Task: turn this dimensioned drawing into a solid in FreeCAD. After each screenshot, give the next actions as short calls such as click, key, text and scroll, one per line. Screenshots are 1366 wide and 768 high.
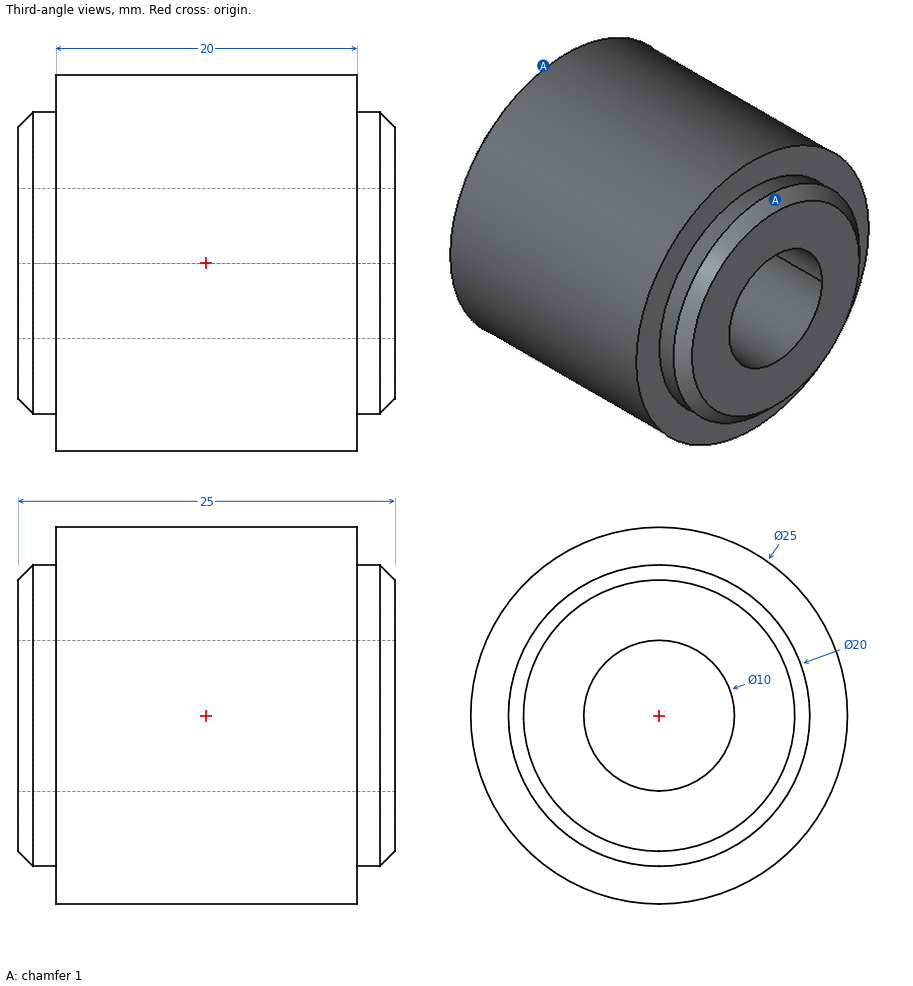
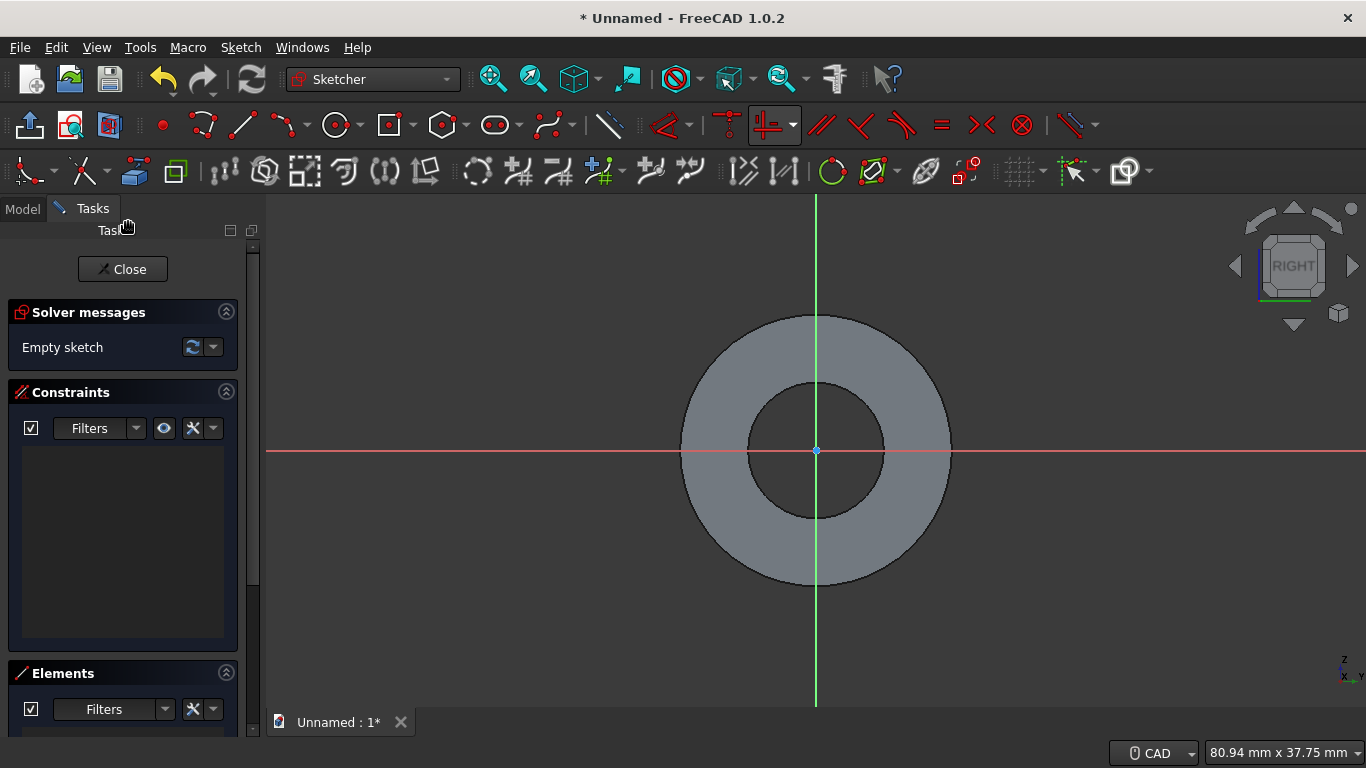
key(g)
key(c)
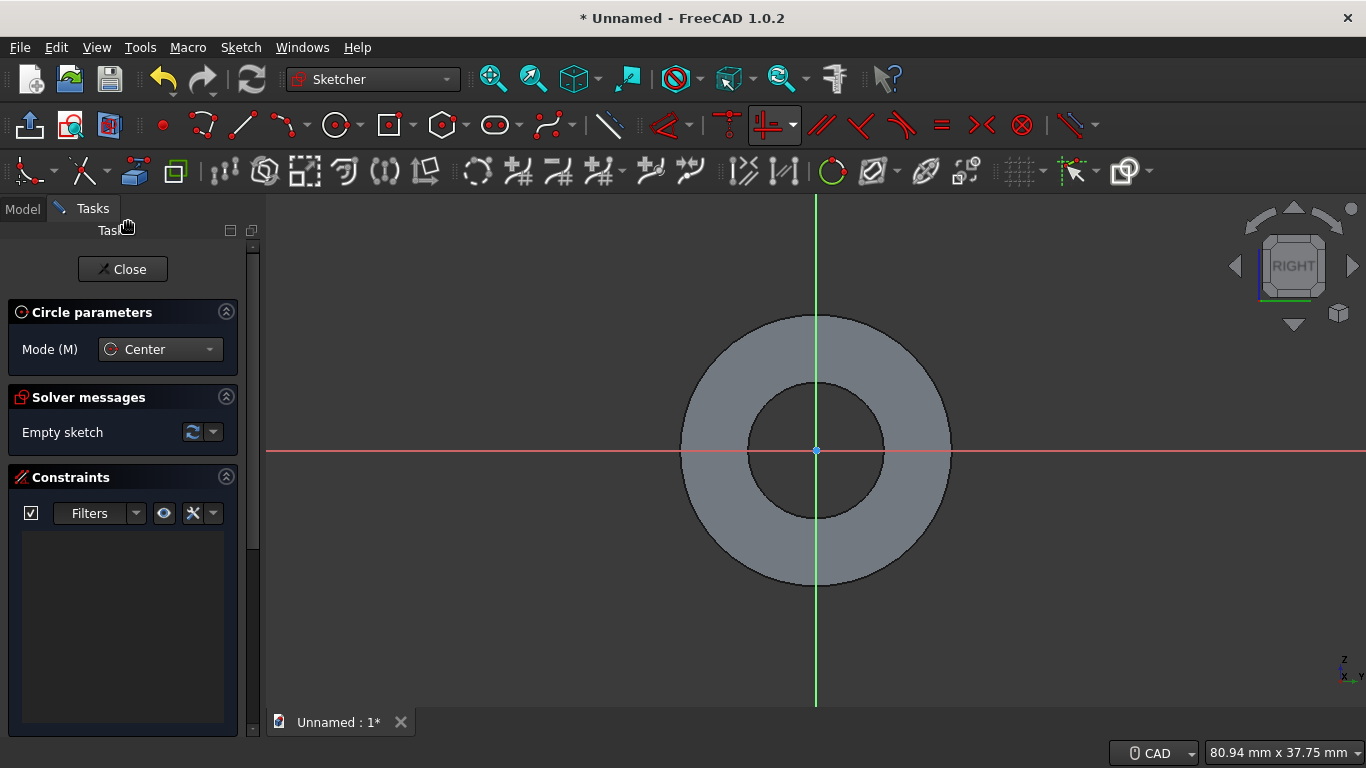
click(816, 450)
move(936, 330)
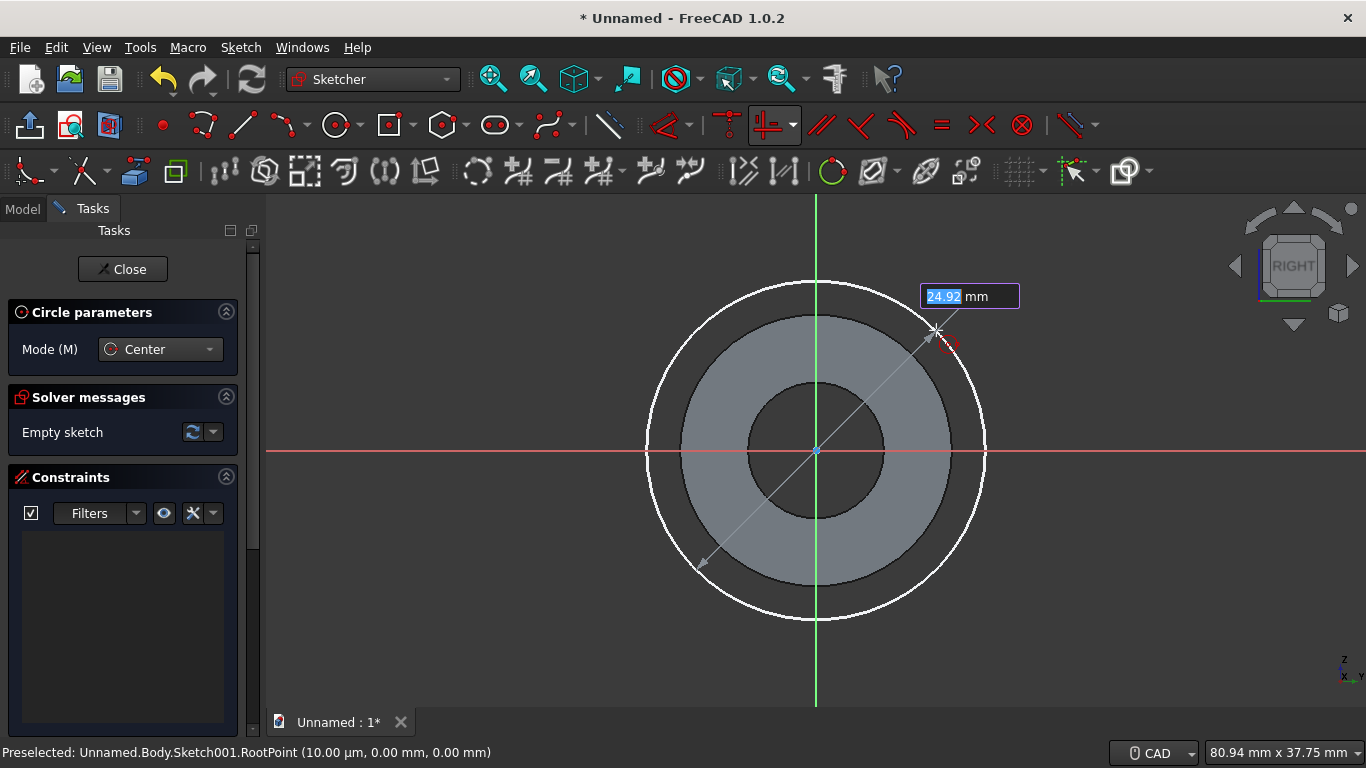
text(25)
key(Return)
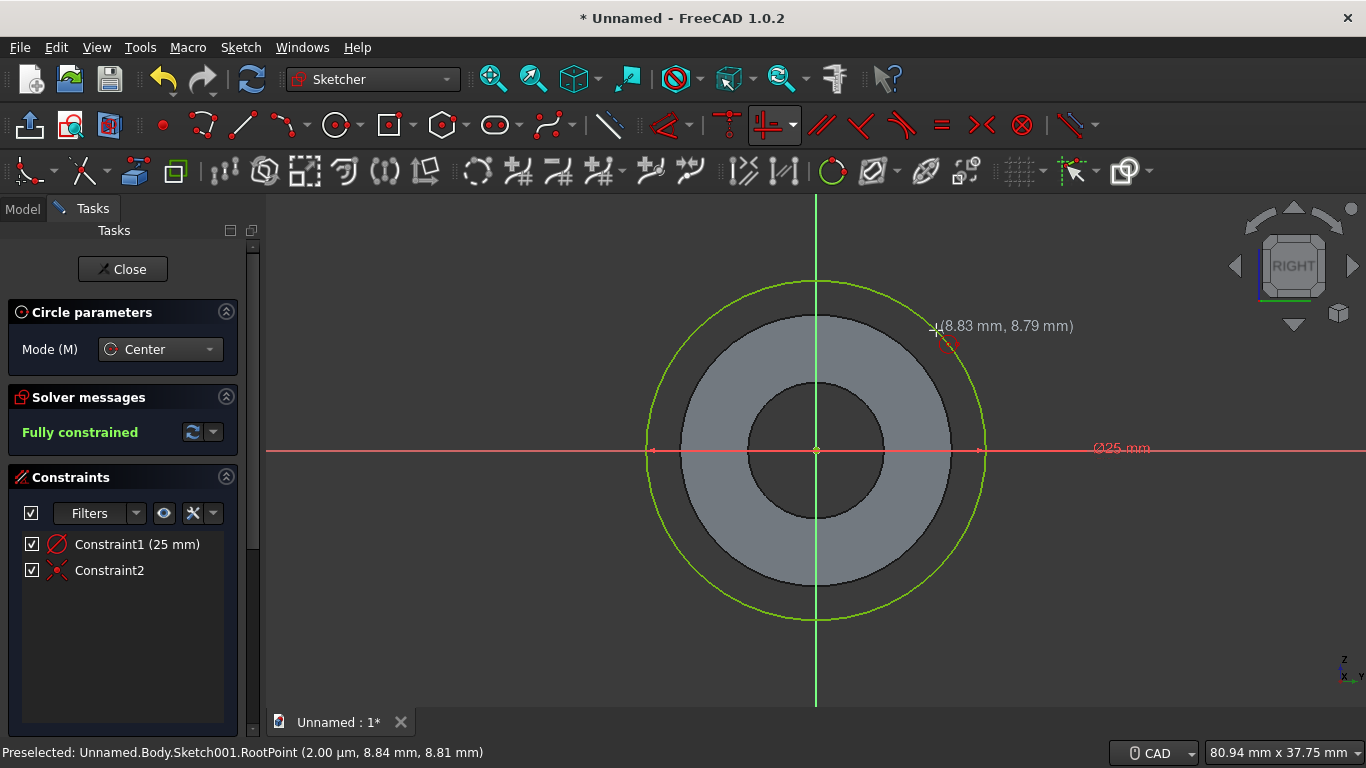
click(816, 450)
move(912, 354)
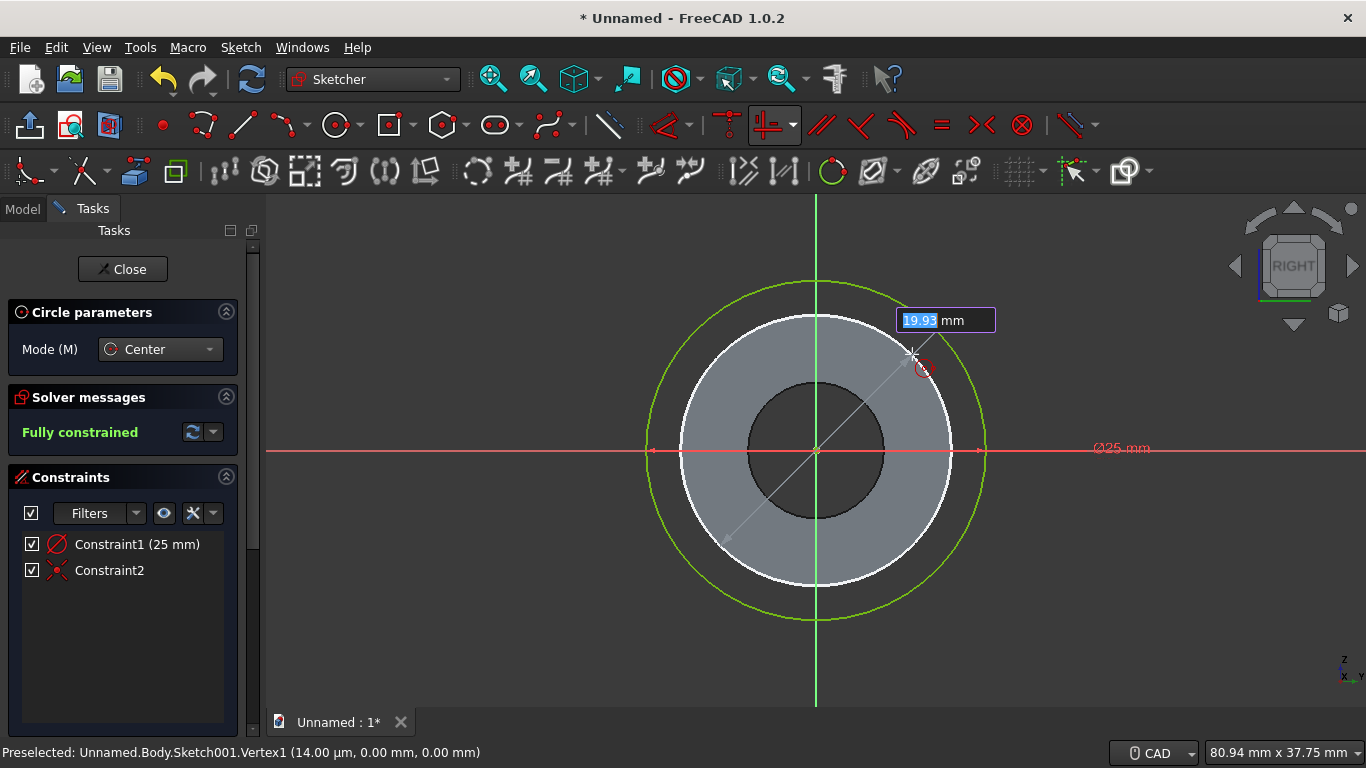
text(20)
key(Return)
key(Escape)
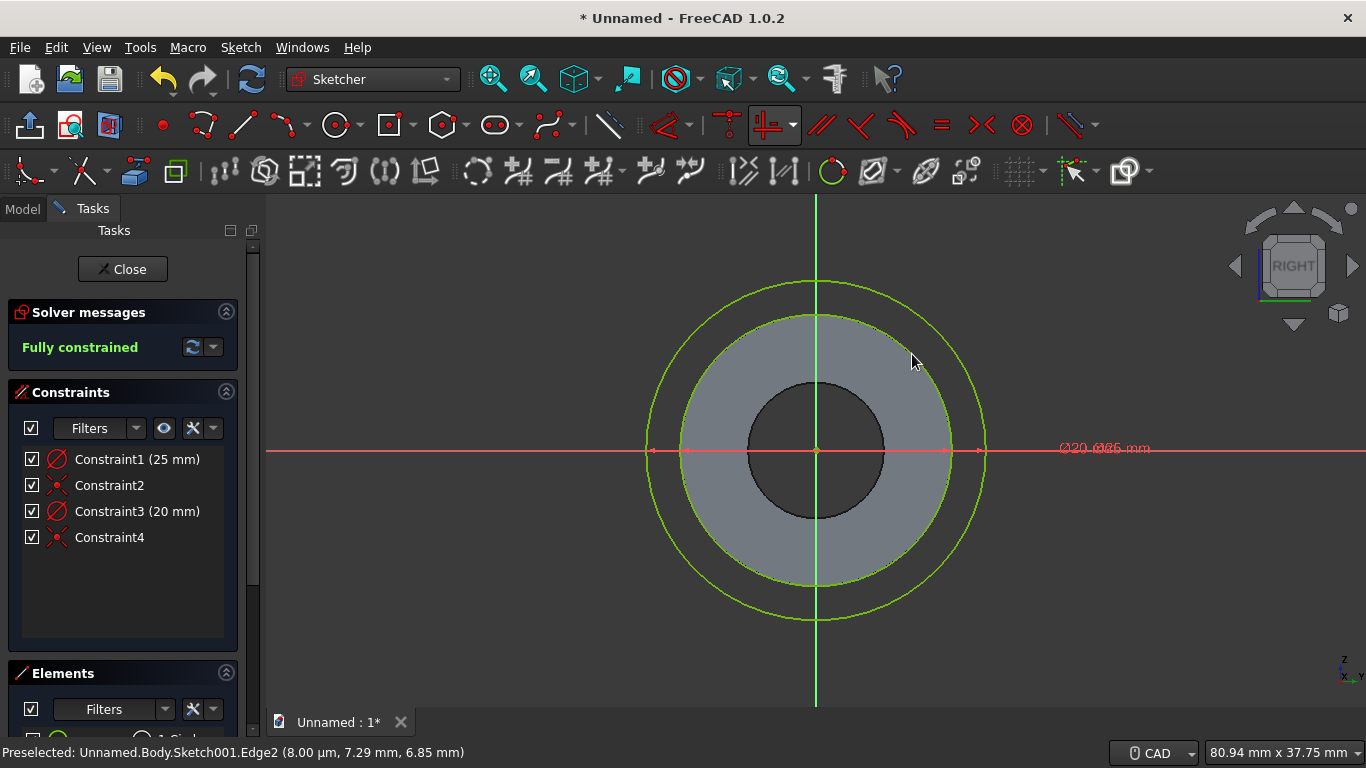
click(123, 269)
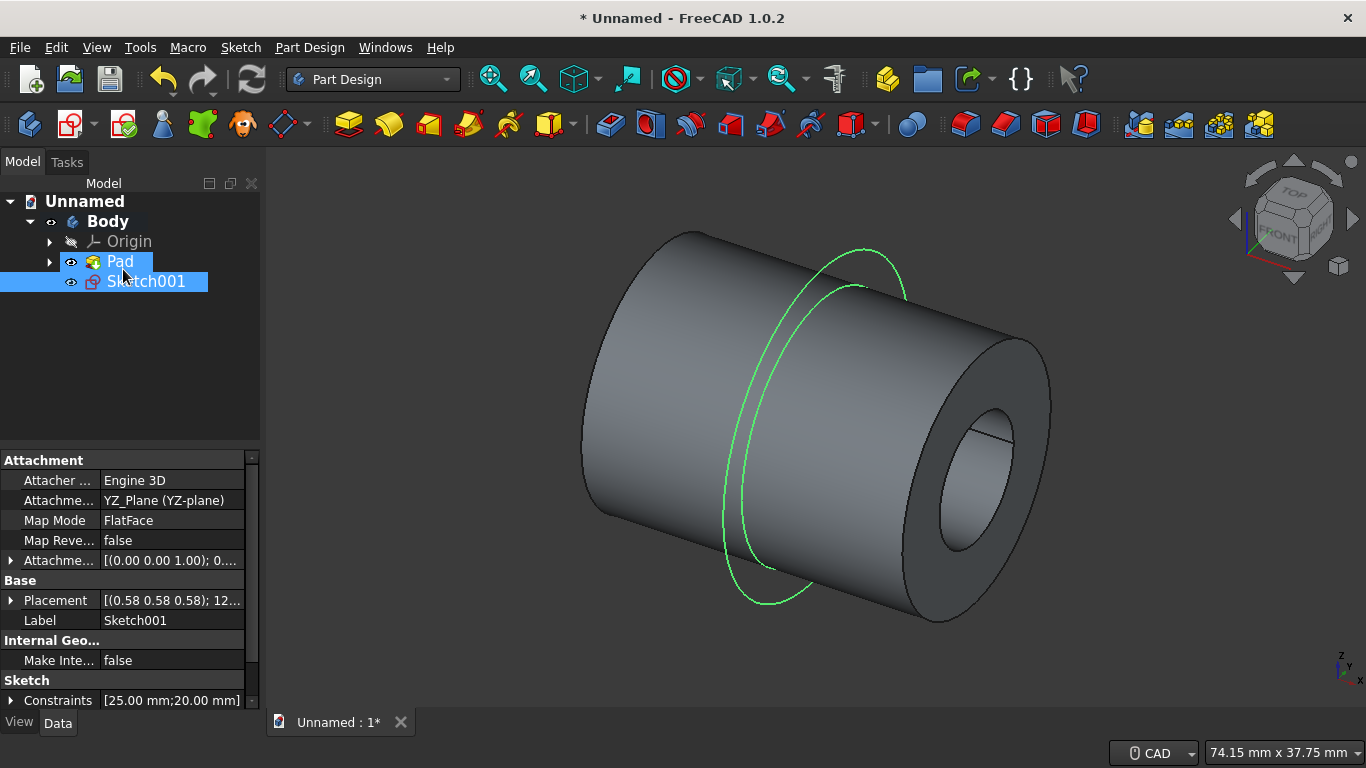
click(350, 124)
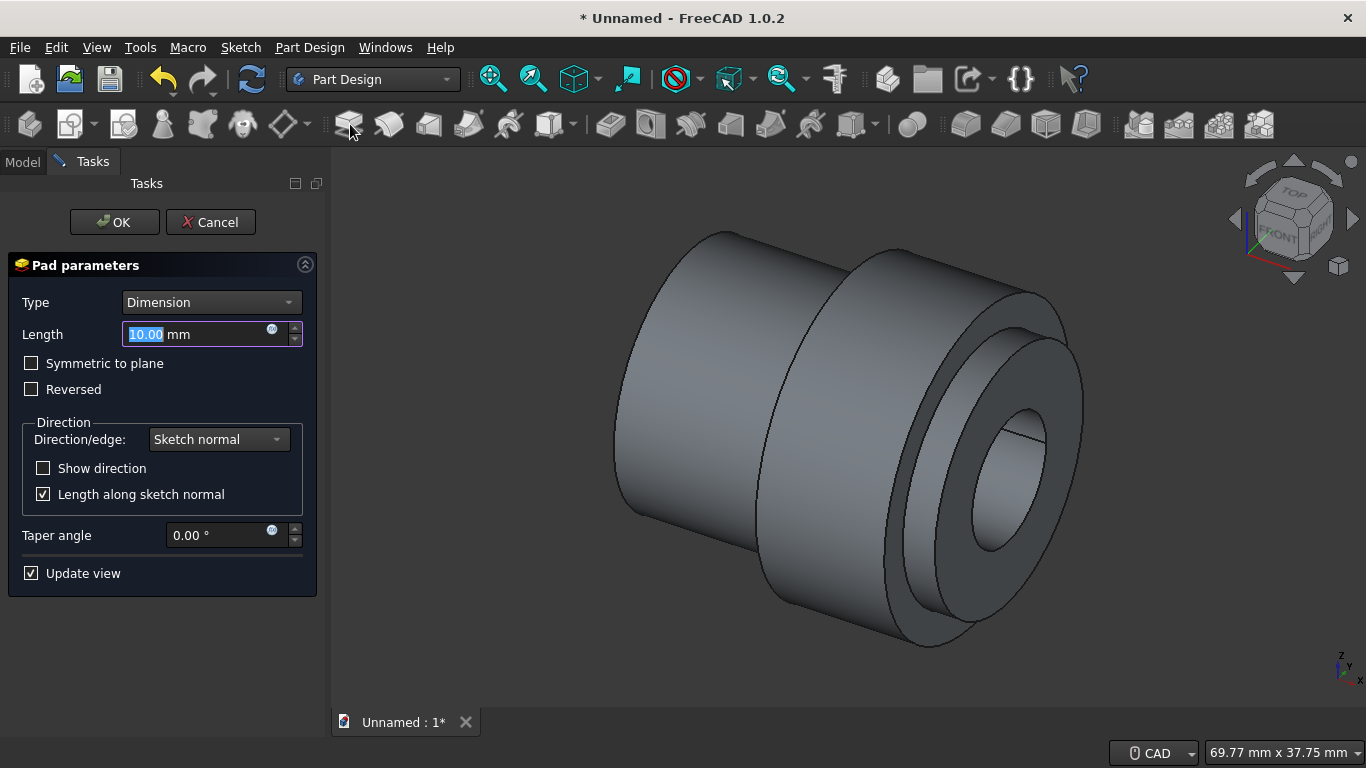
text(20)
key(Tab)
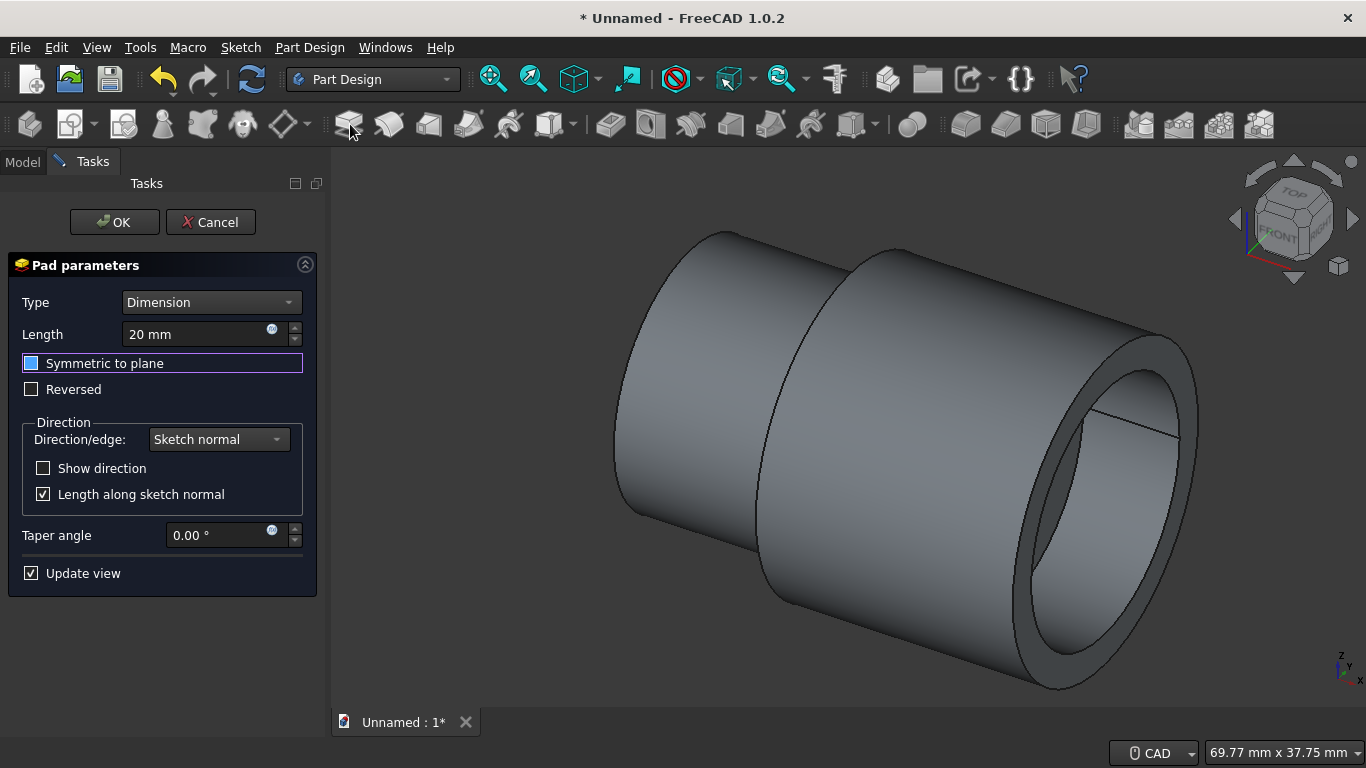
click(30, 363)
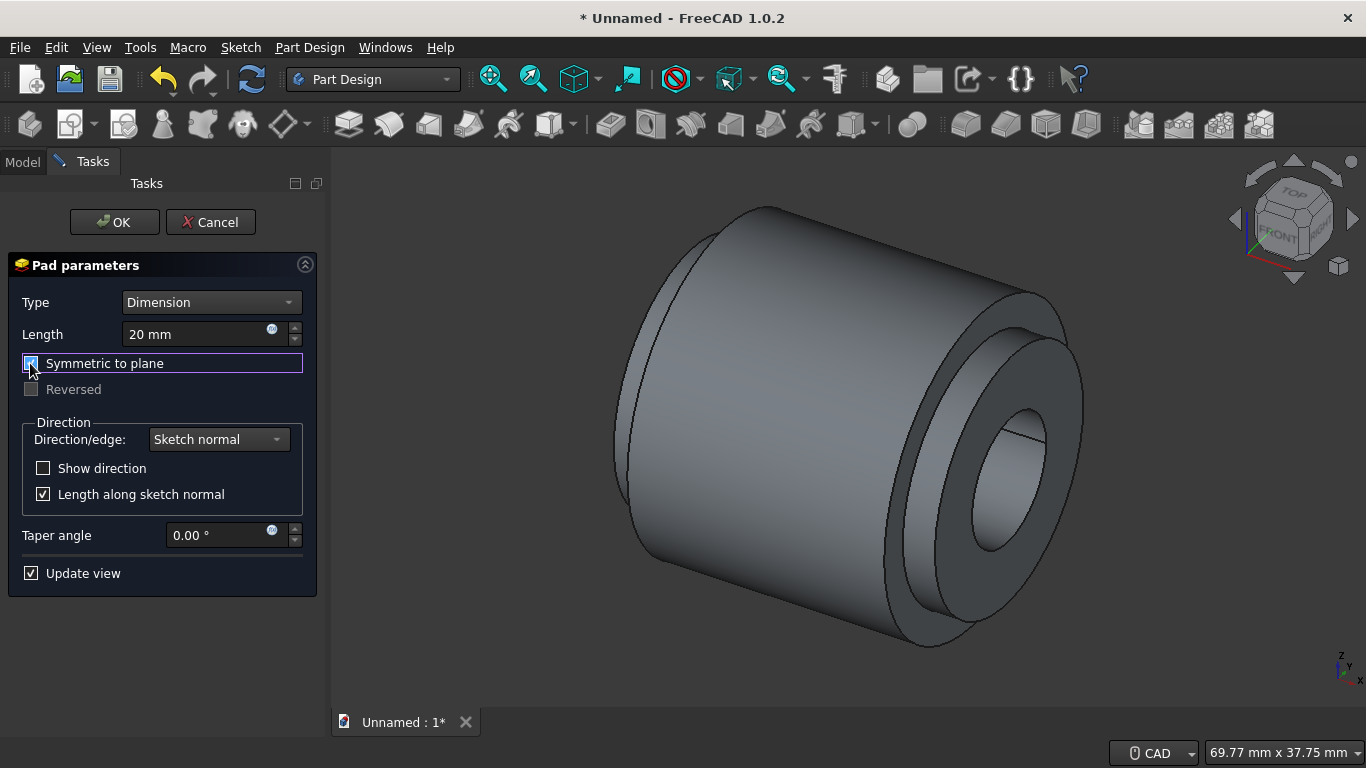
click(115, 222)